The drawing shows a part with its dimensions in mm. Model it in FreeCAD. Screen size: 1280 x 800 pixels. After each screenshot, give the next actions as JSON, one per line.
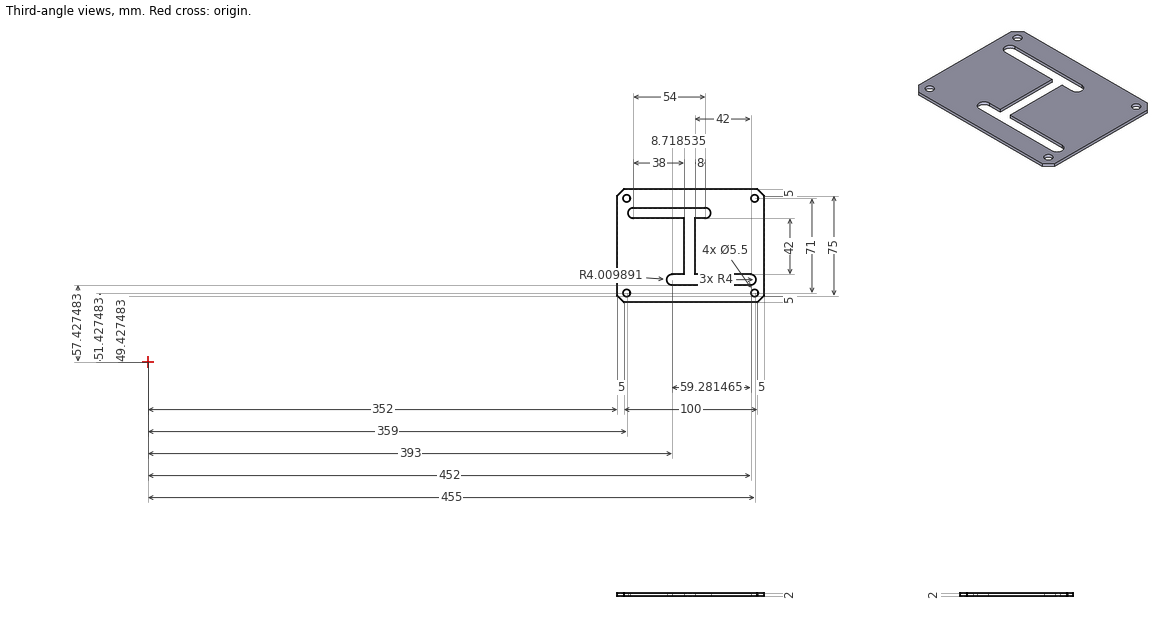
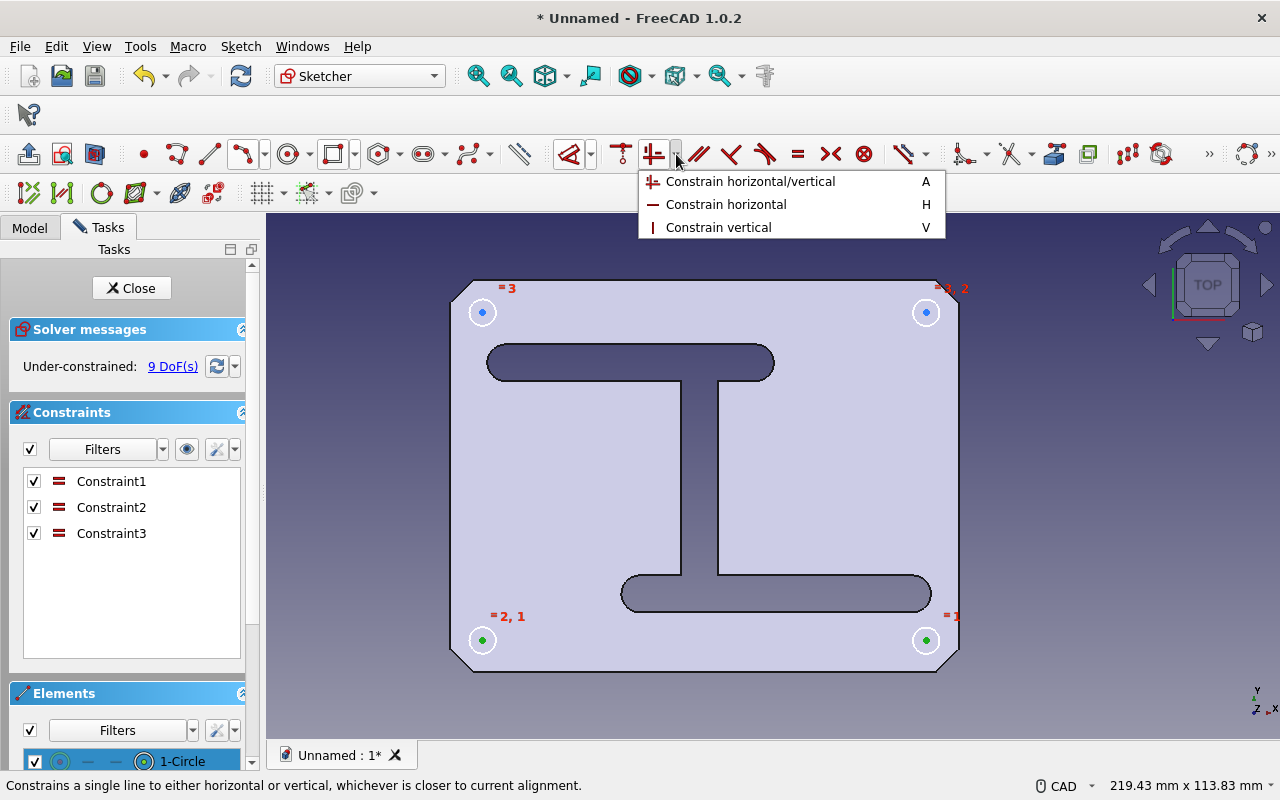
{"action": "left_click", "coordinate": [792, 204]}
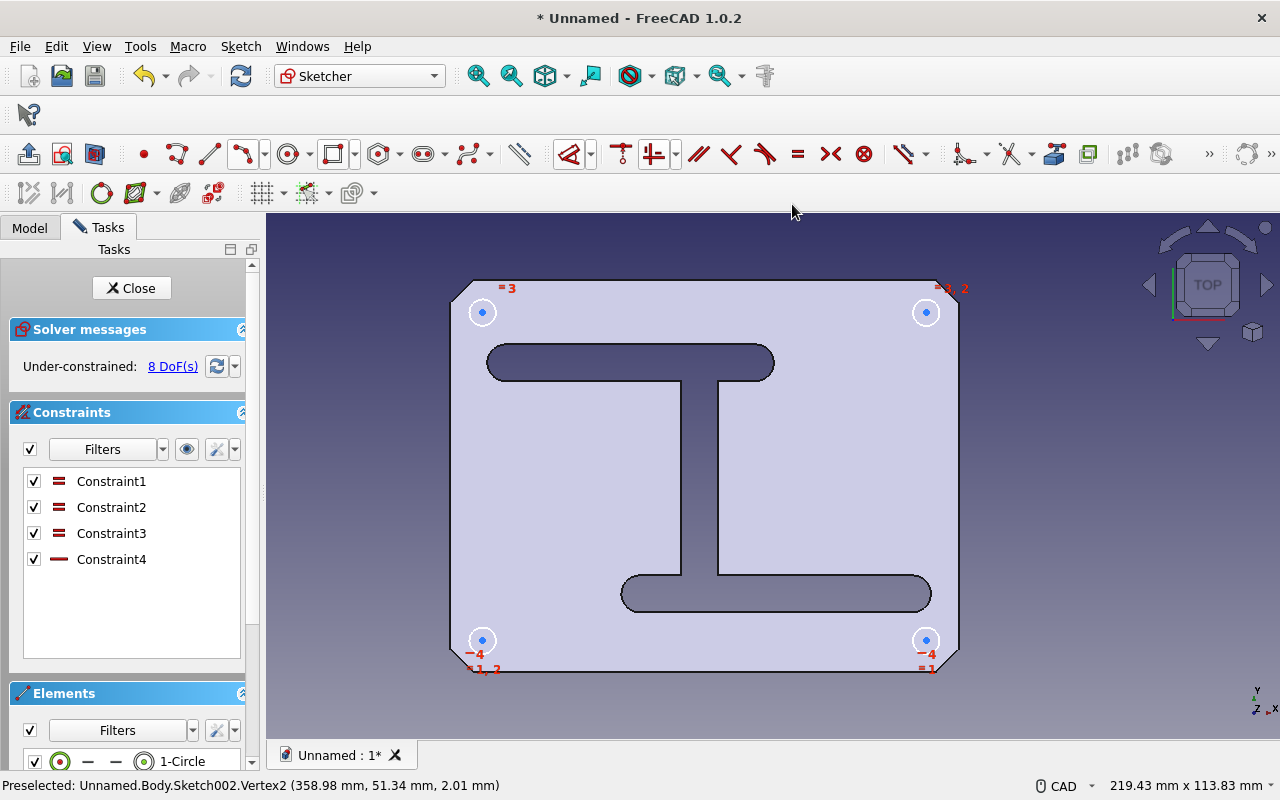
{"action": "left_click", "coordinate": [926, 641]}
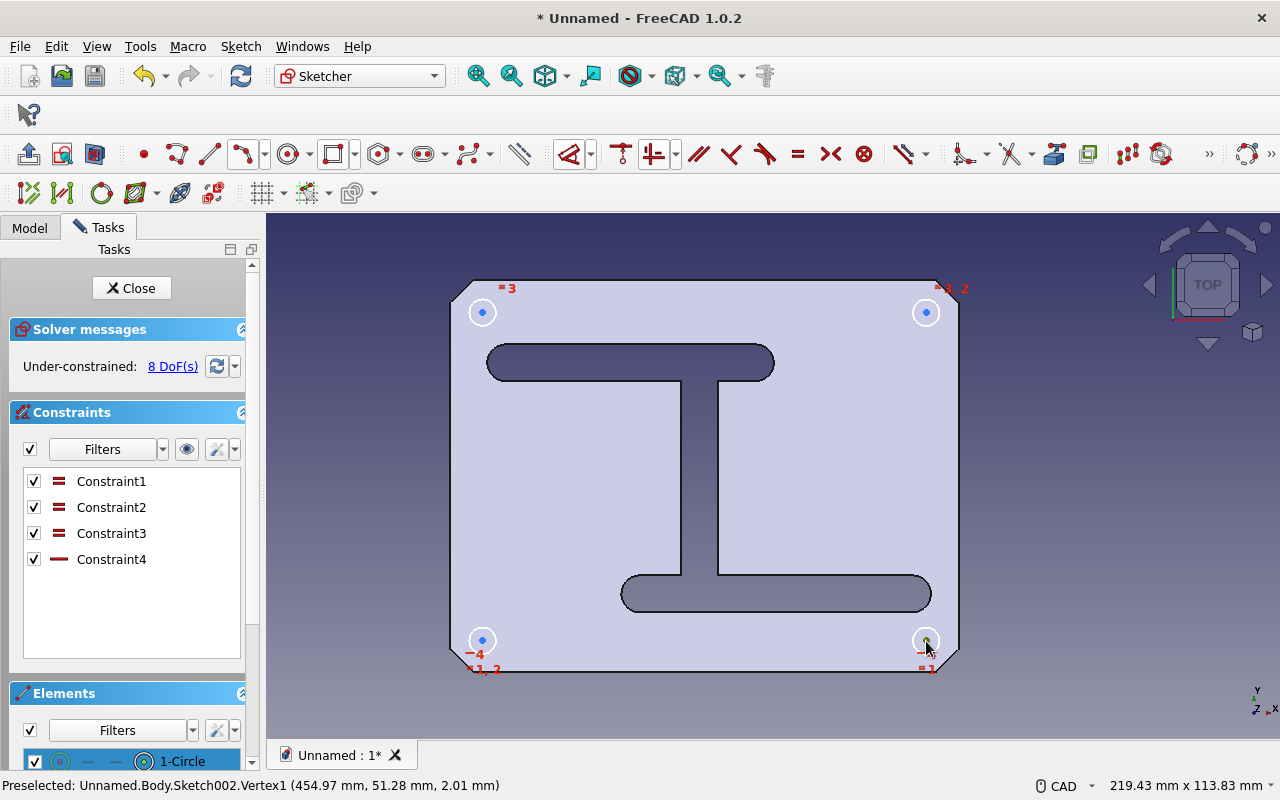
{"action": "left_click", "coordinate": [926, 313]}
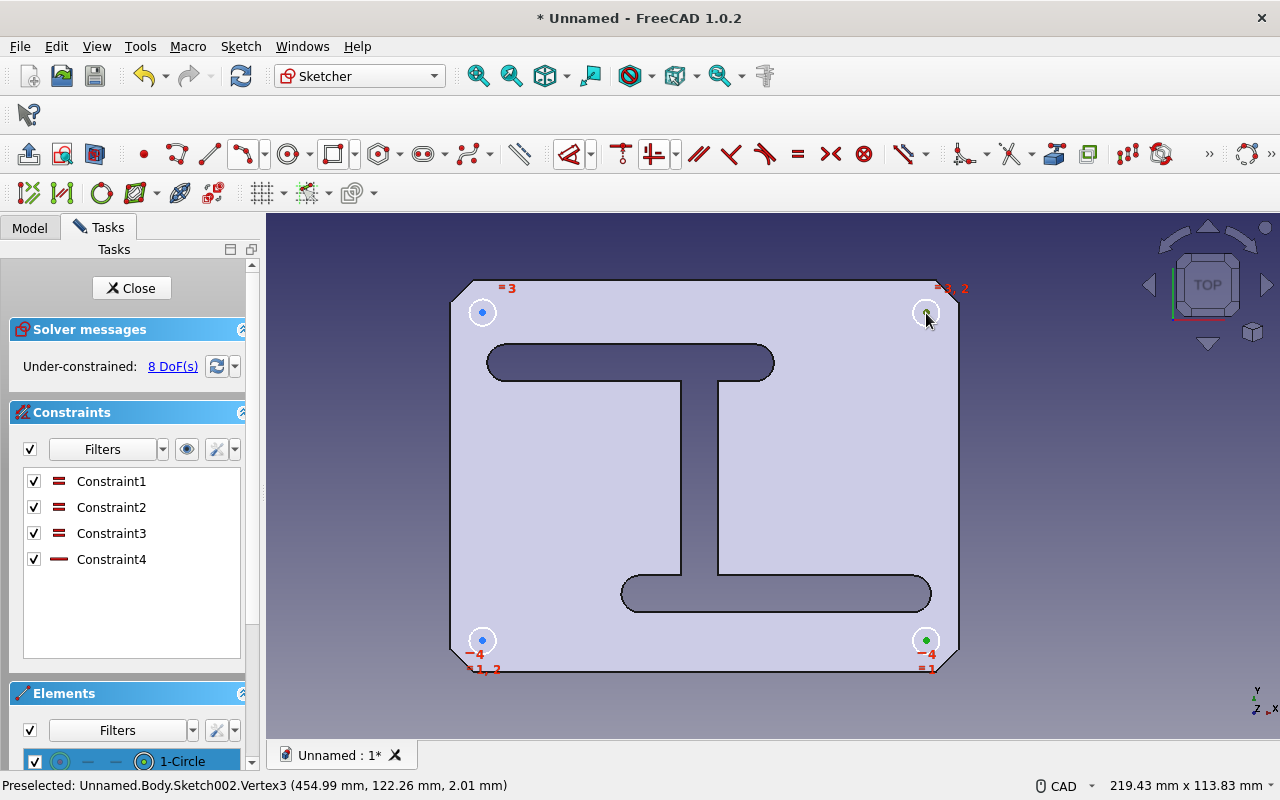
{"action": "key", "text": "v"}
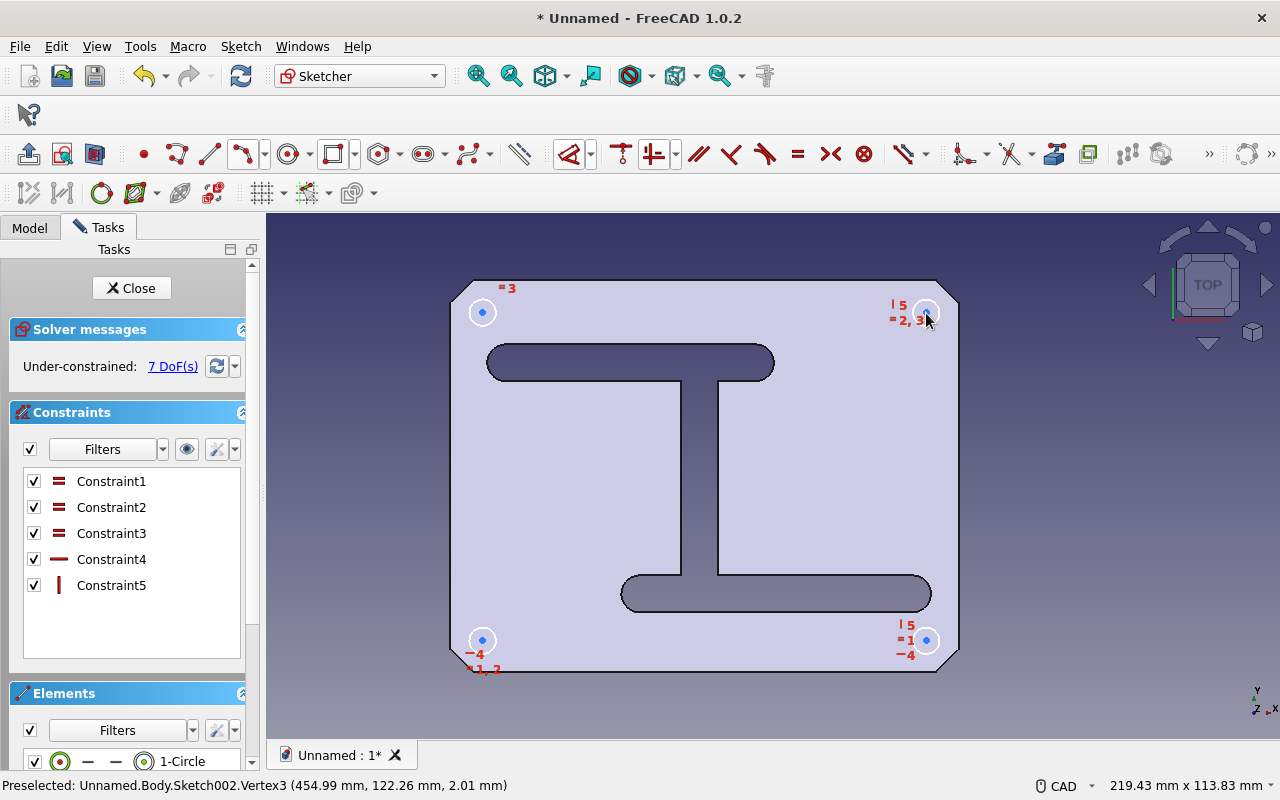
{"action": "left_click", "coordinate": [483, 641]}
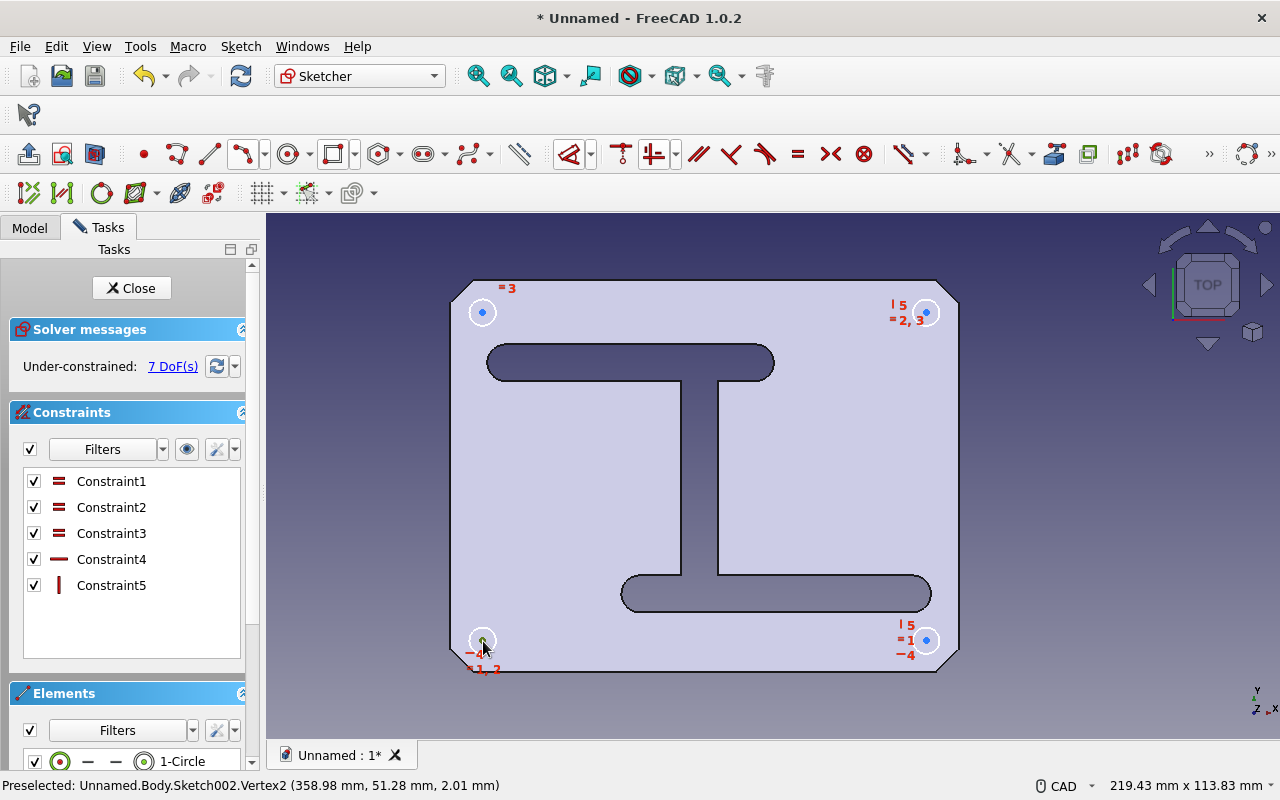
{"action": "left_click", "coordinate": [483, 313]}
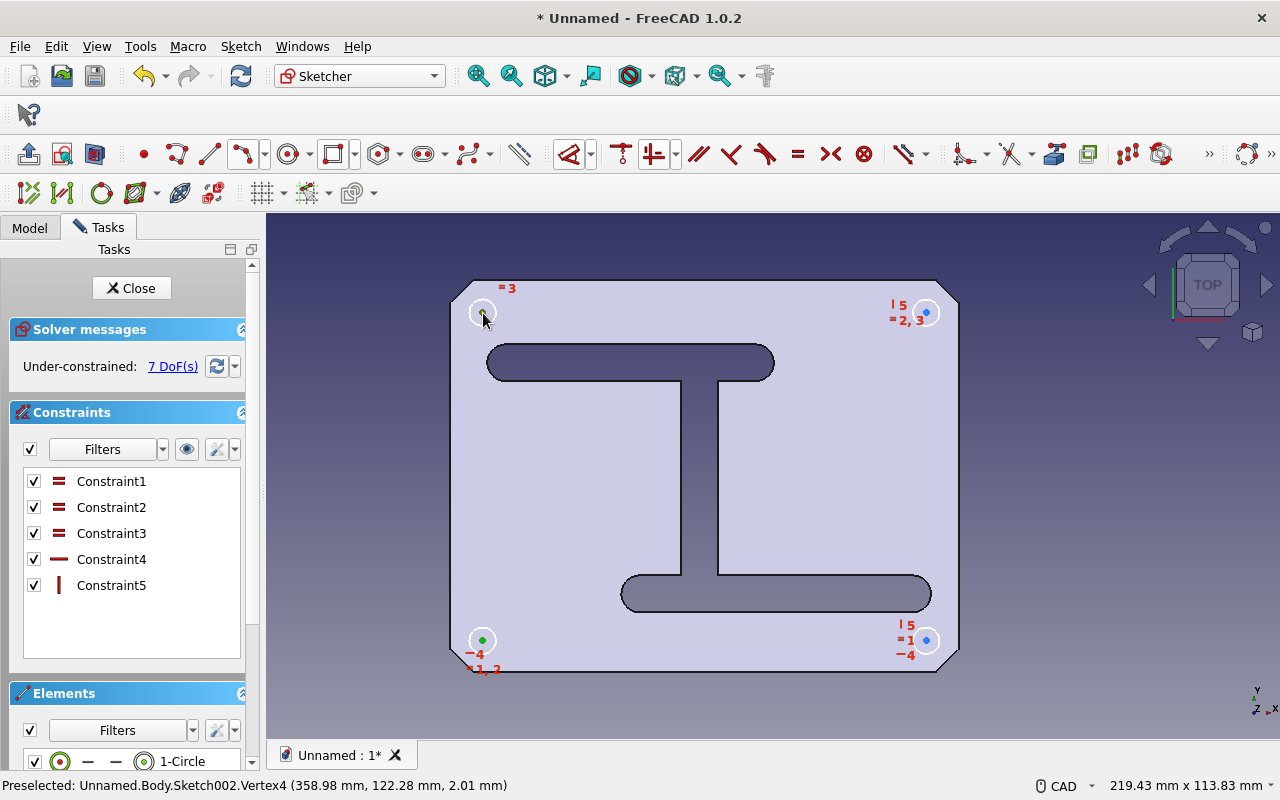
{"action": "left_click", "coordinate": [676, 154]}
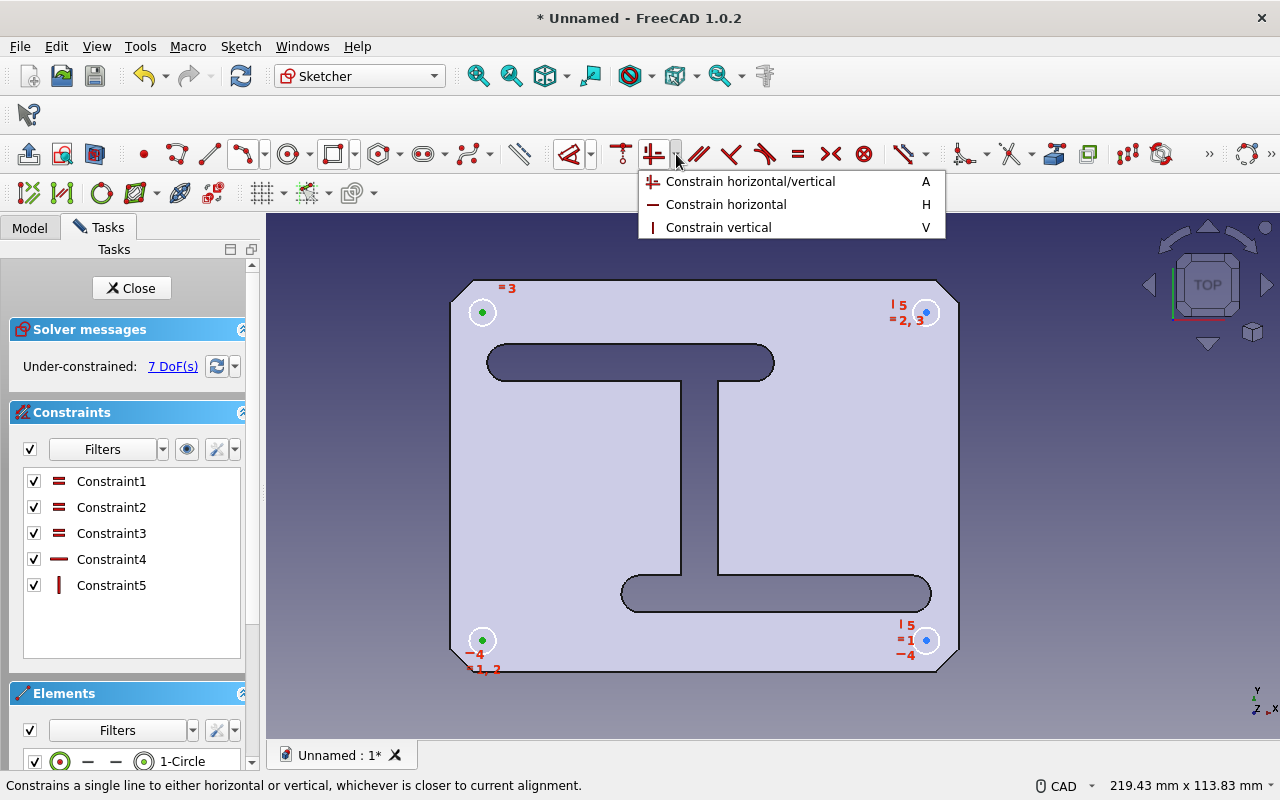
{"action": "left_click", "coordinate": [792, 228]}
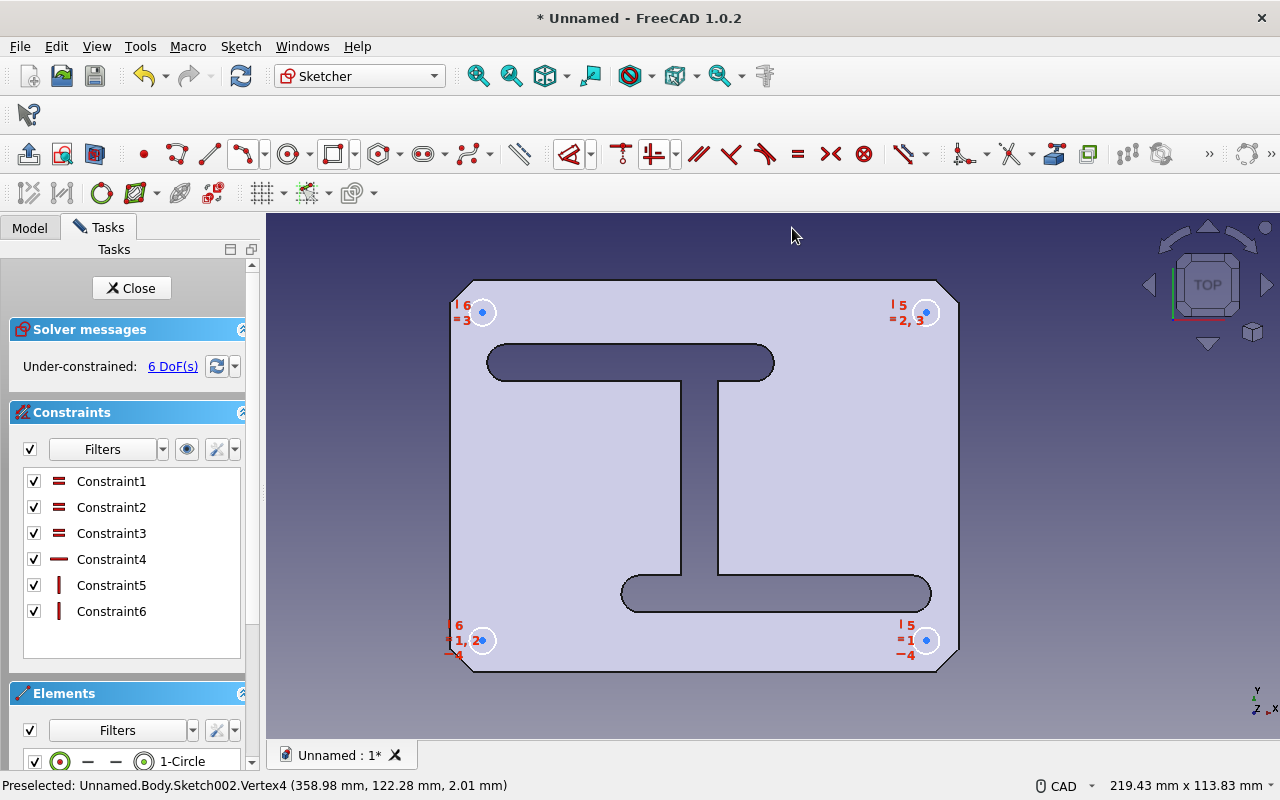
{"action": "left_click", "coordinate": [926, 313]}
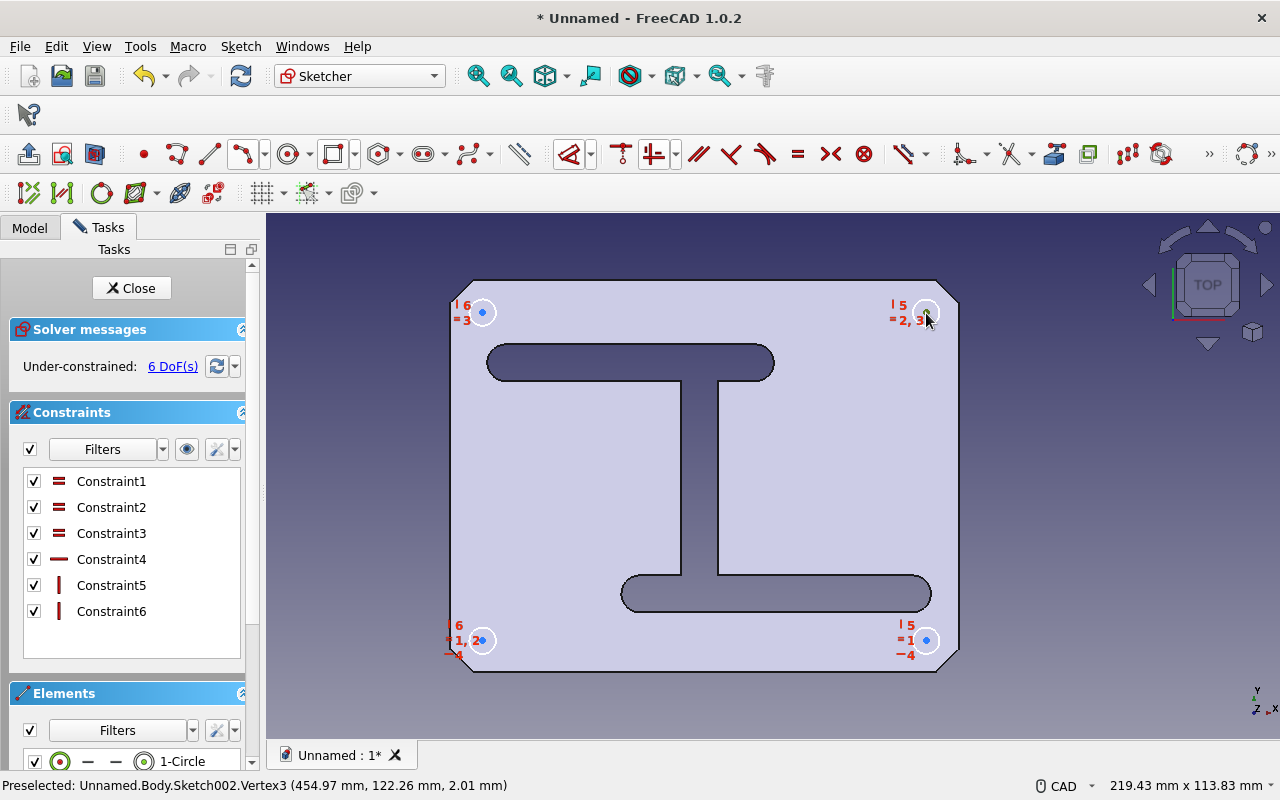
{"action": "left_click", "coordinate": [483, 313]}